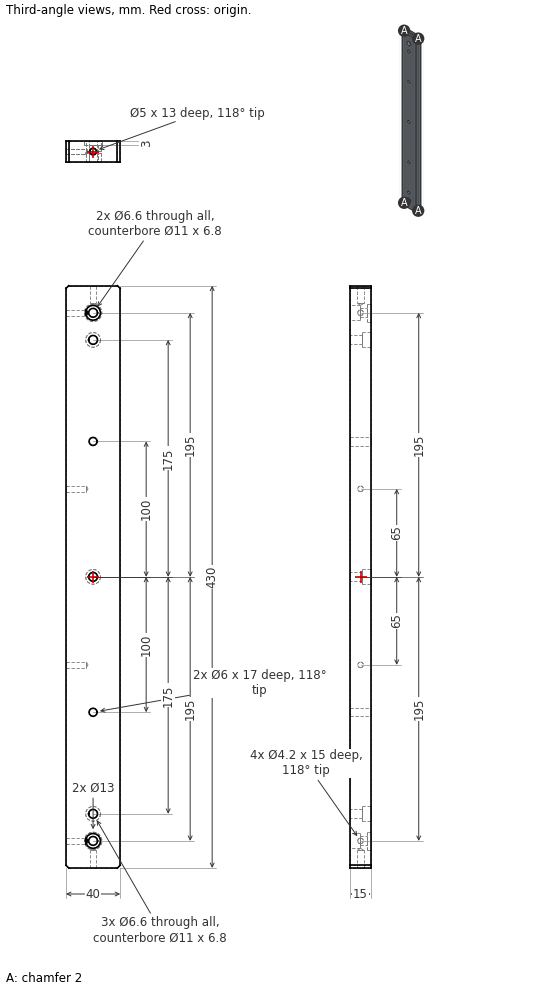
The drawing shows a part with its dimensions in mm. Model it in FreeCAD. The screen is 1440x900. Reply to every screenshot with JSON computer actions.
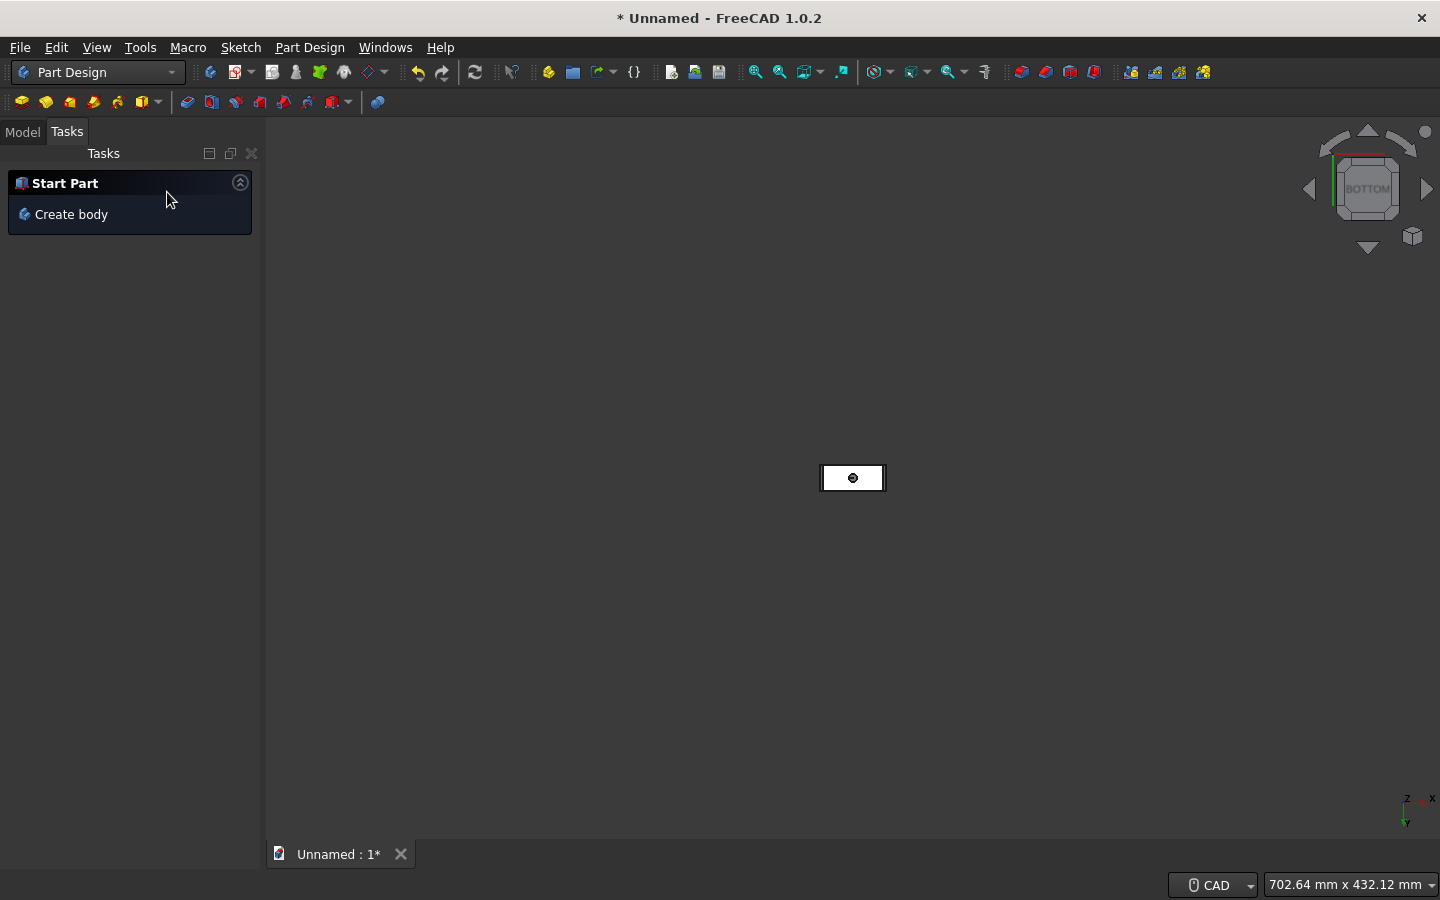
{"action": "left_click", "coordinate": [756, 72]}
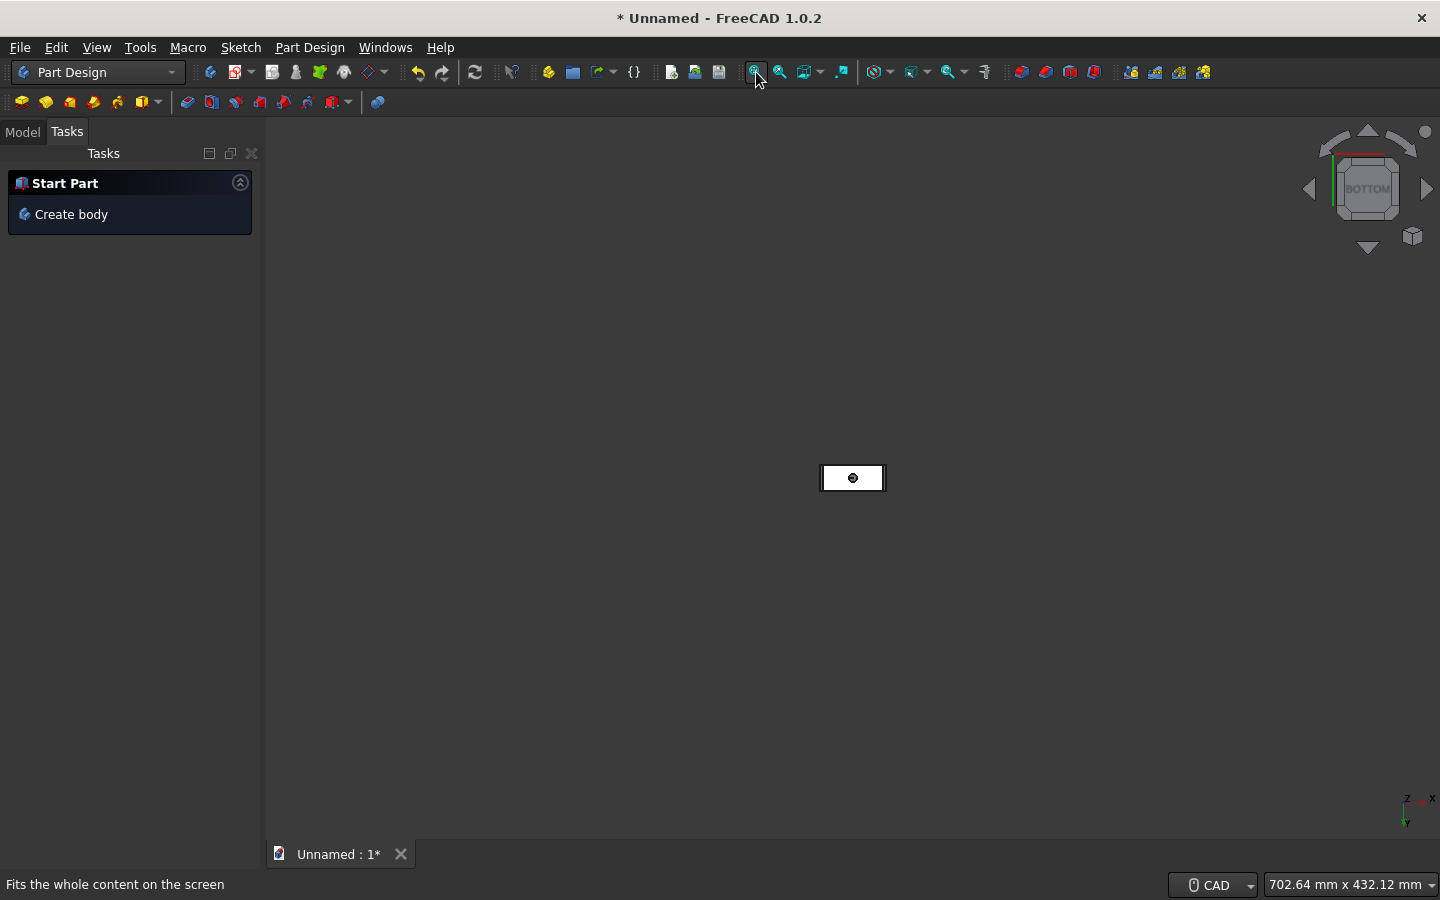
{"action": "key", "text": "0"}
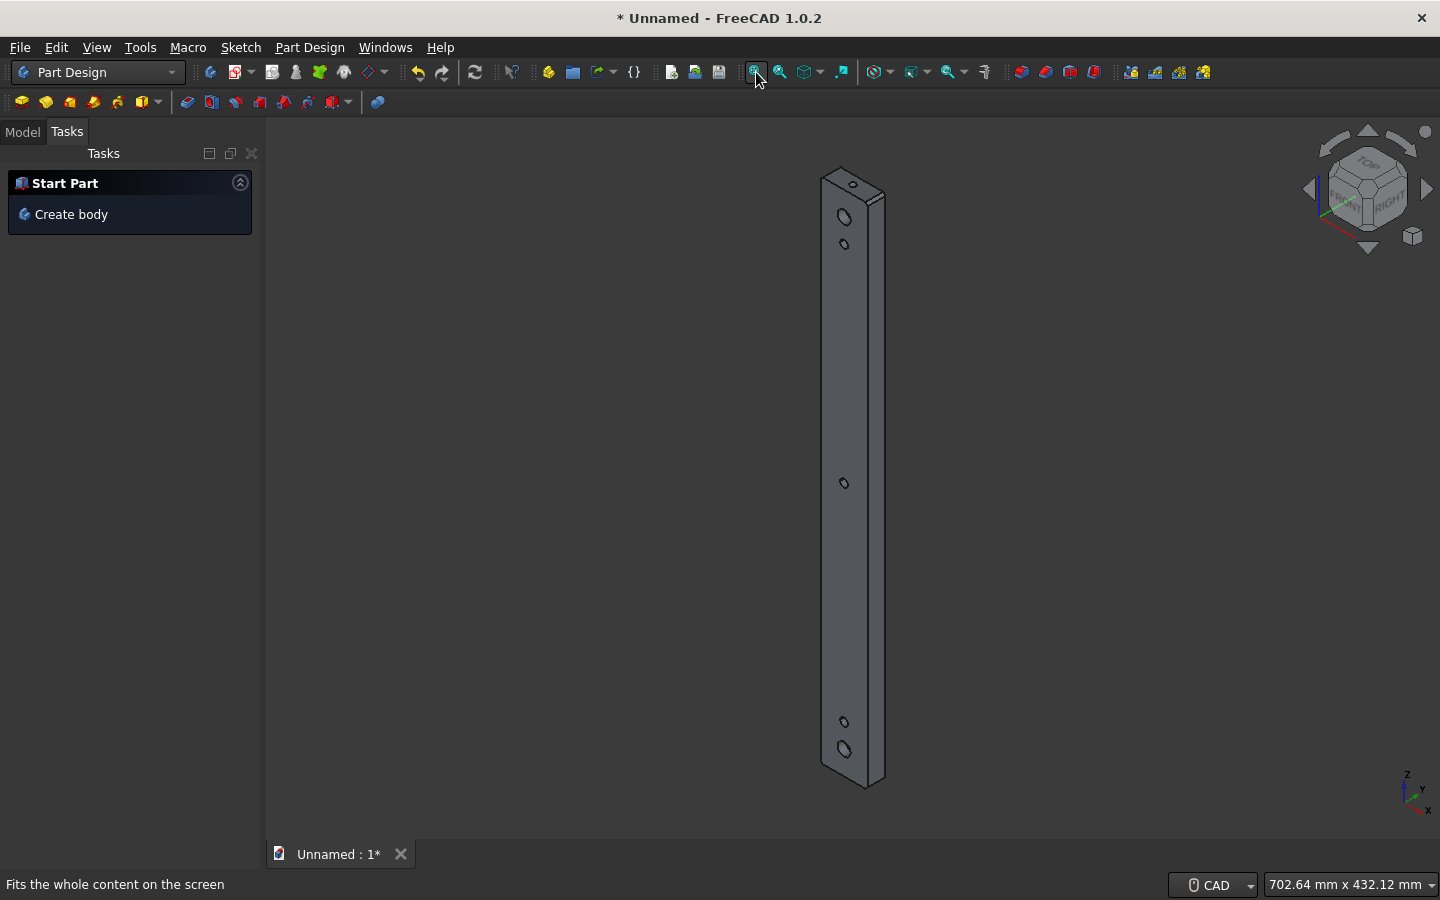
{"action": "left_click", "coordinate": [844, 315]}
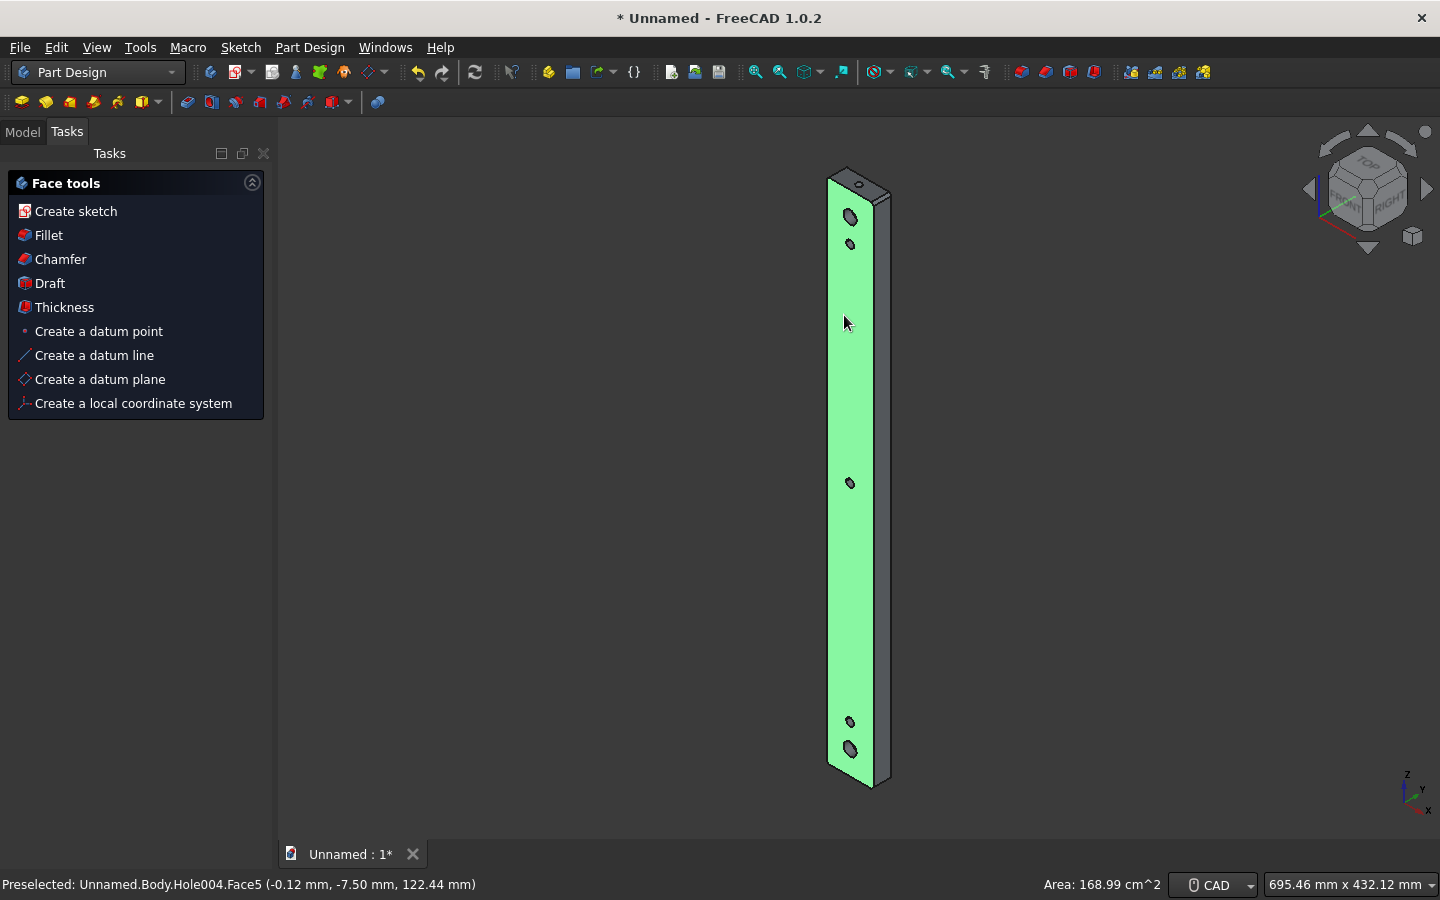
{"action": "left_click", "coordinate": [236, 72]}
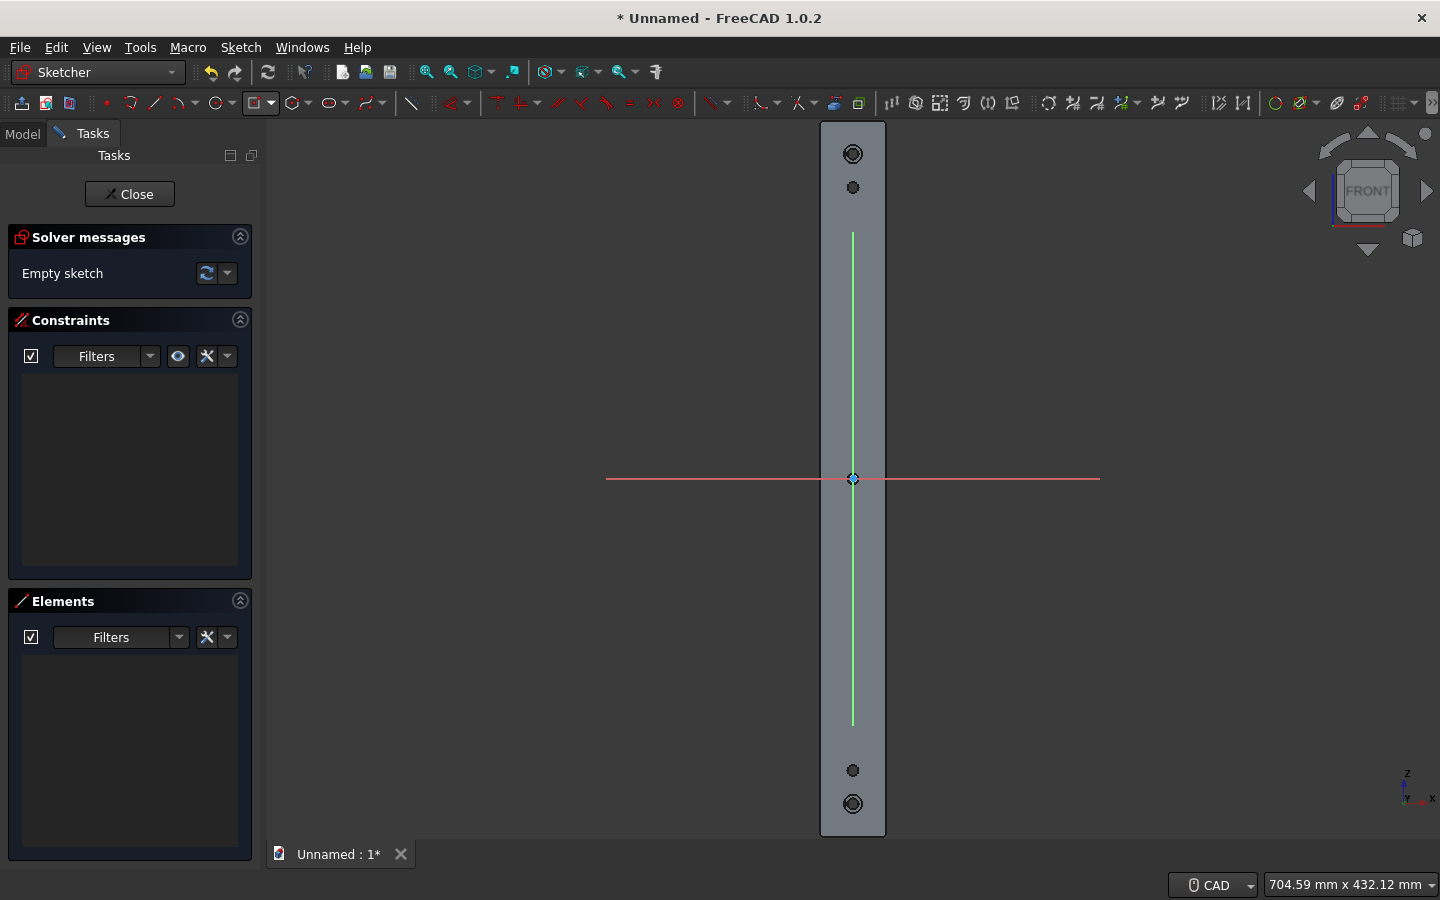
{"action": "scroll", "coordinate": [992, 479], "scroll_direction": "up", "scroll_amount": 2}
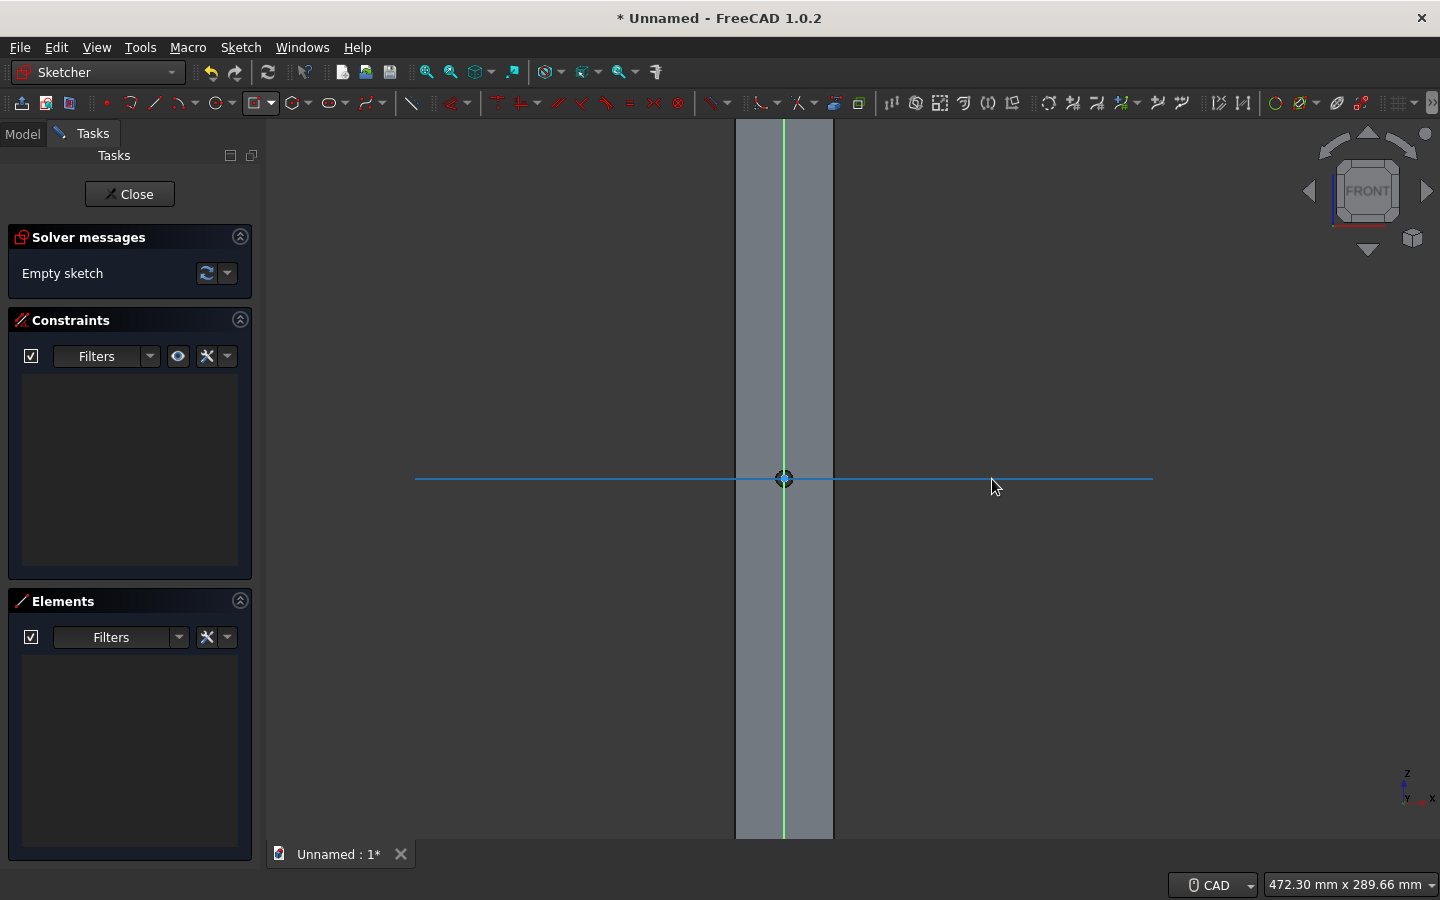
{"action": "left_click", "coordinate": [216, 104]}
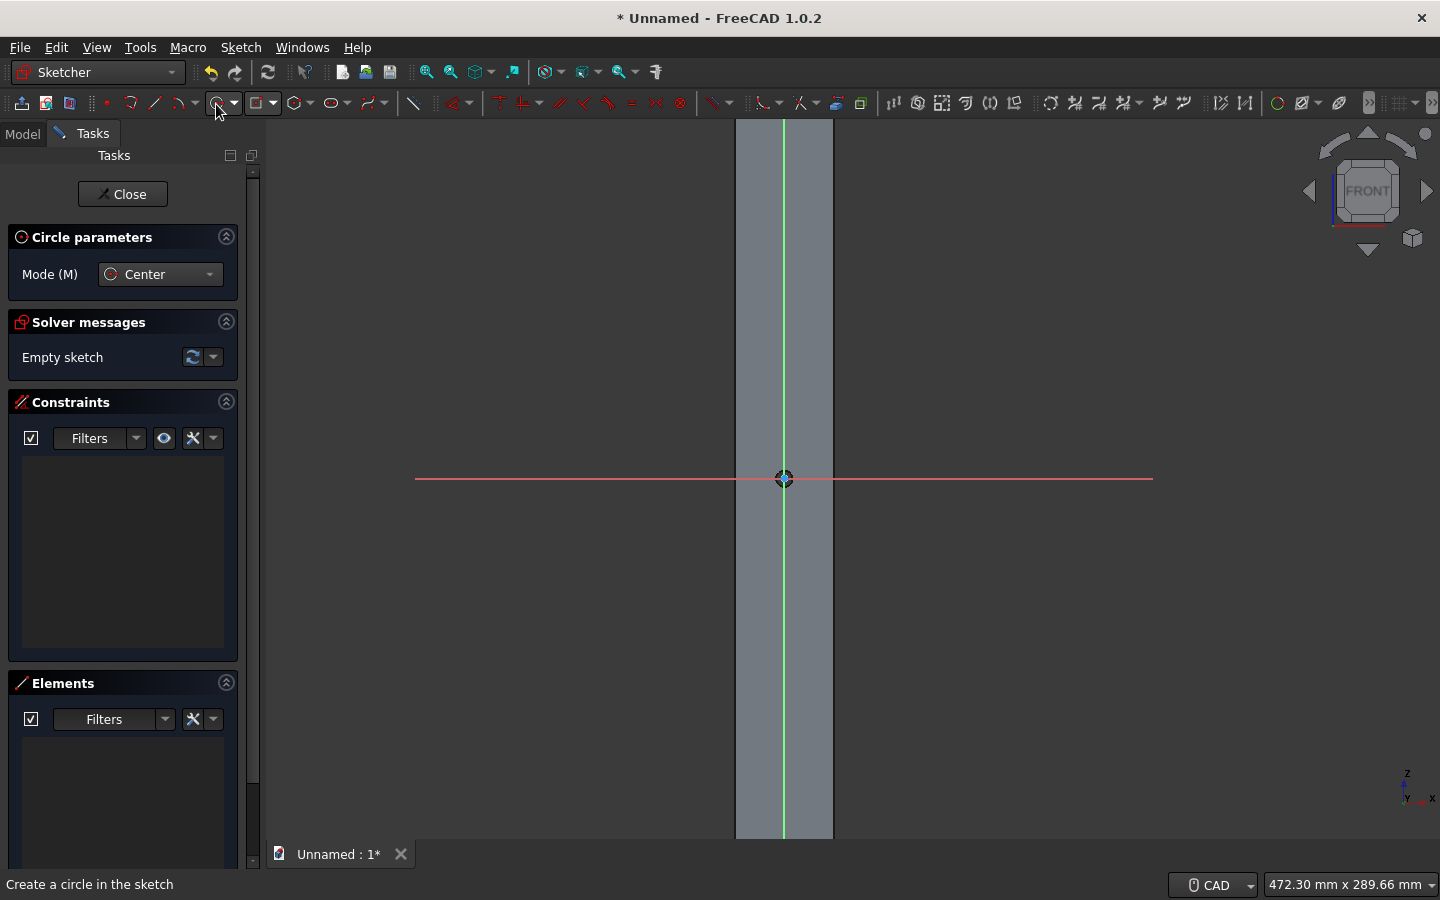
{"action": "scroll", "coordinate": [784, 727], "scroll_direction": "up", "scroll_amount": 6}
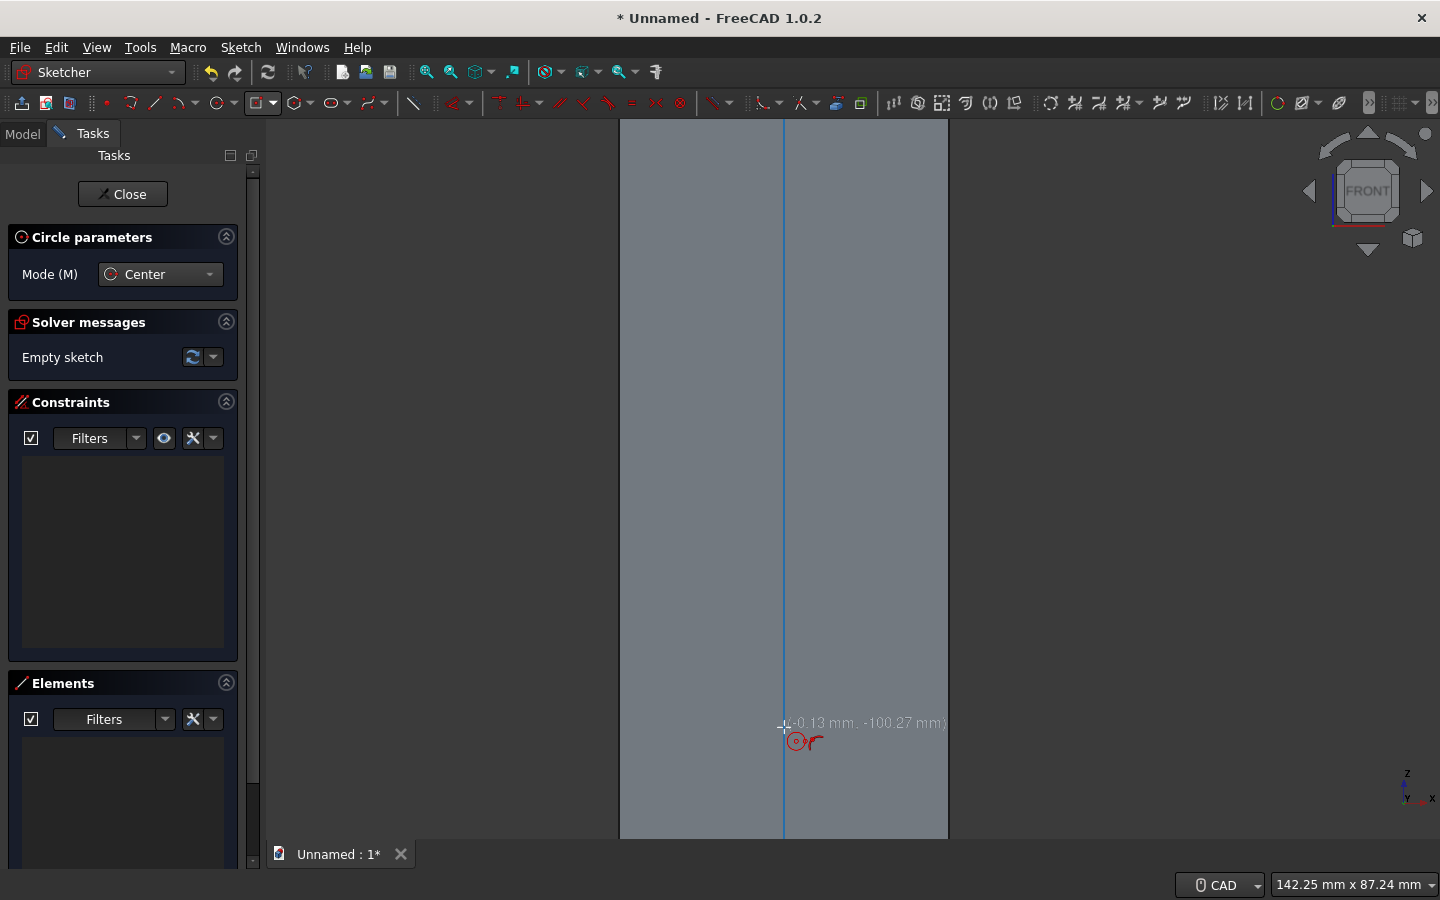
{"action": "left_click", "coordinate": [784, 726]}
{"action": "left_click", "coordinate": [802, 709]}